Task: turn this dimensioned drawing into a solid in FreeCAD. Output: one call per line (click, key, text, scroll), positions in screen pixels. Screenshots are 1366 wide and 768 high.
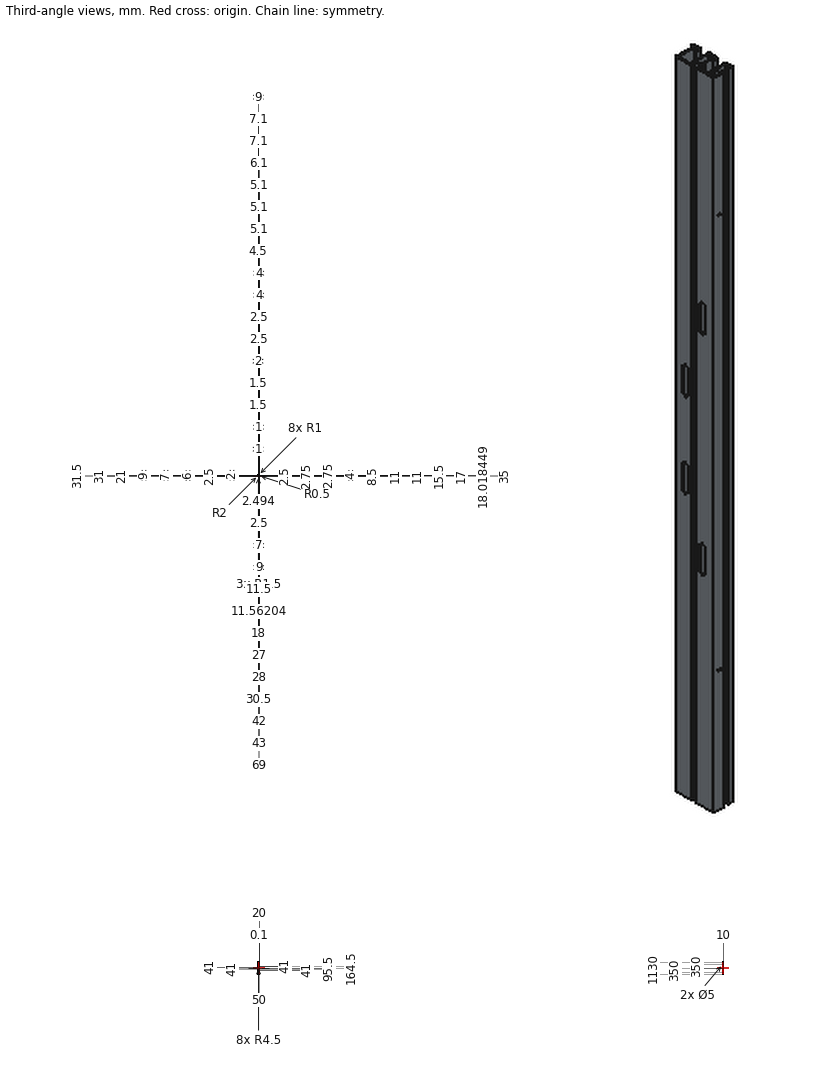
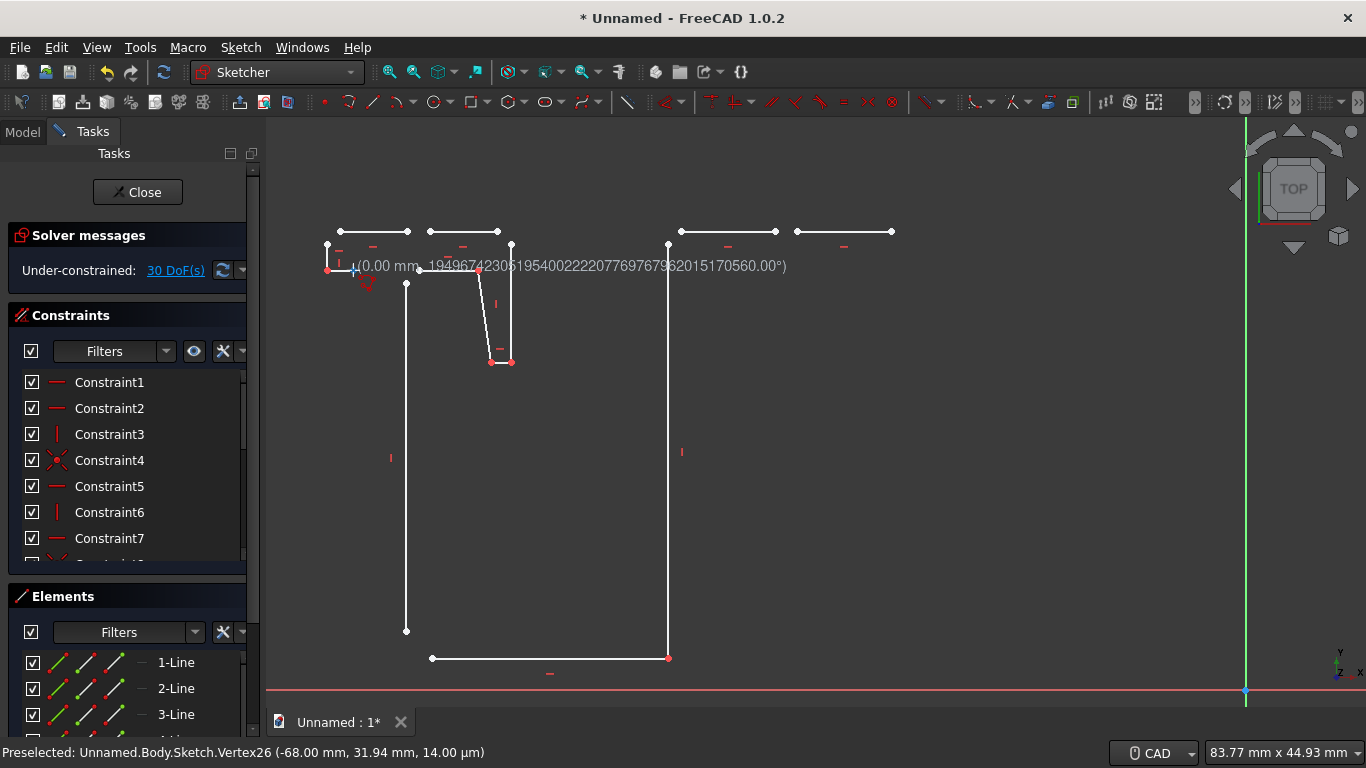
click(366, 283)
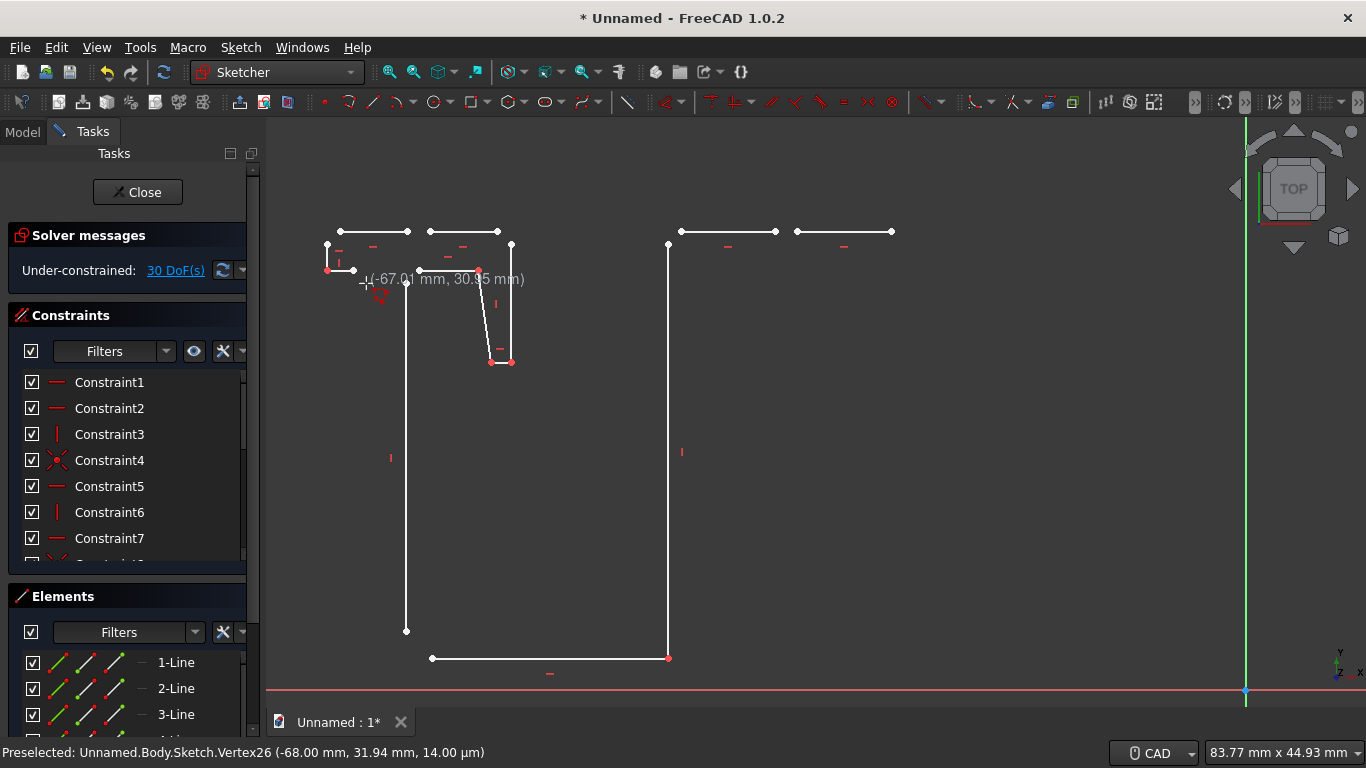
scroll(669, 313, down, 2)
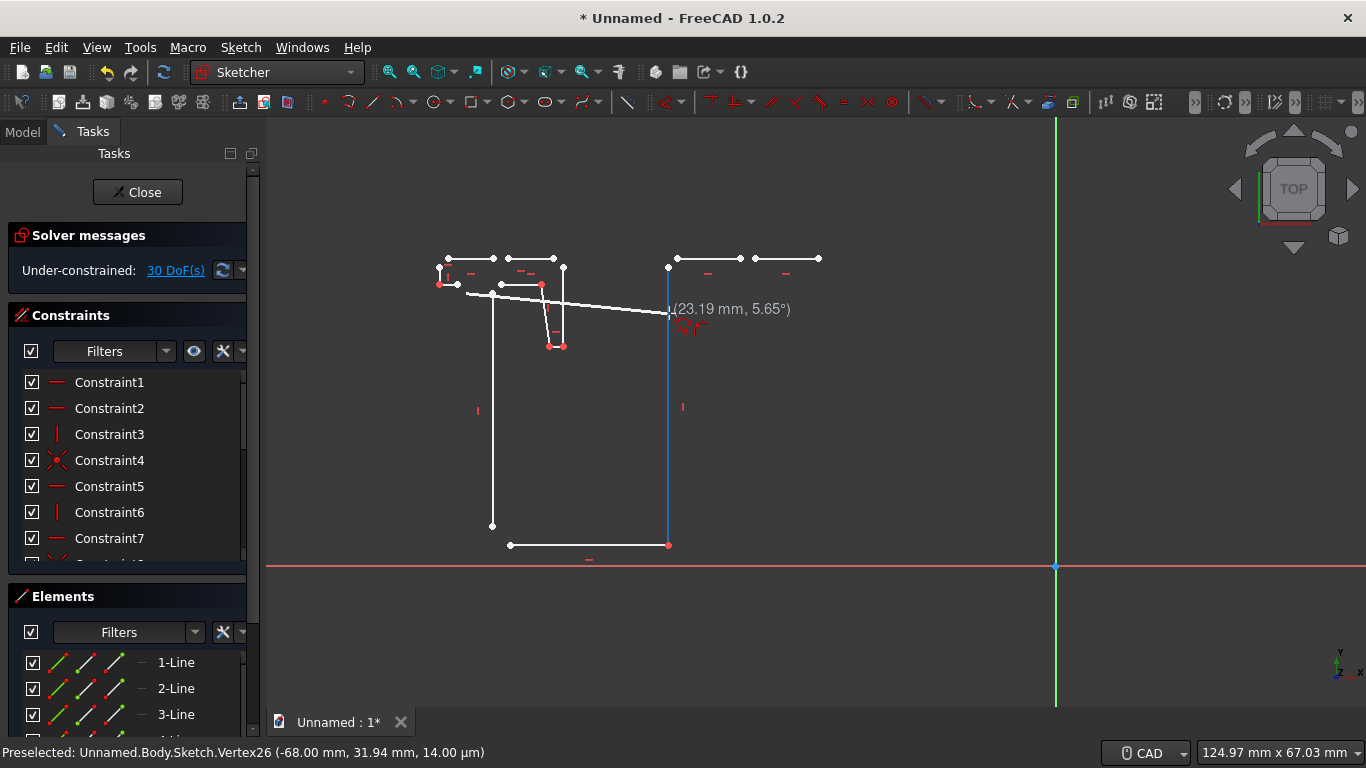
click(466, 566)
click(713, 557)
click(713, 544)
click(691, 544)
click(691, 491)
click(809, 491)
click(809, 544)
click(787, 544)
click(787, 566)
click(1056, 566)
click(1047, 405)
click(1034, 405)
click(1034, 430)
click(955, 430)
click(955, 293)
right_click(955, 293)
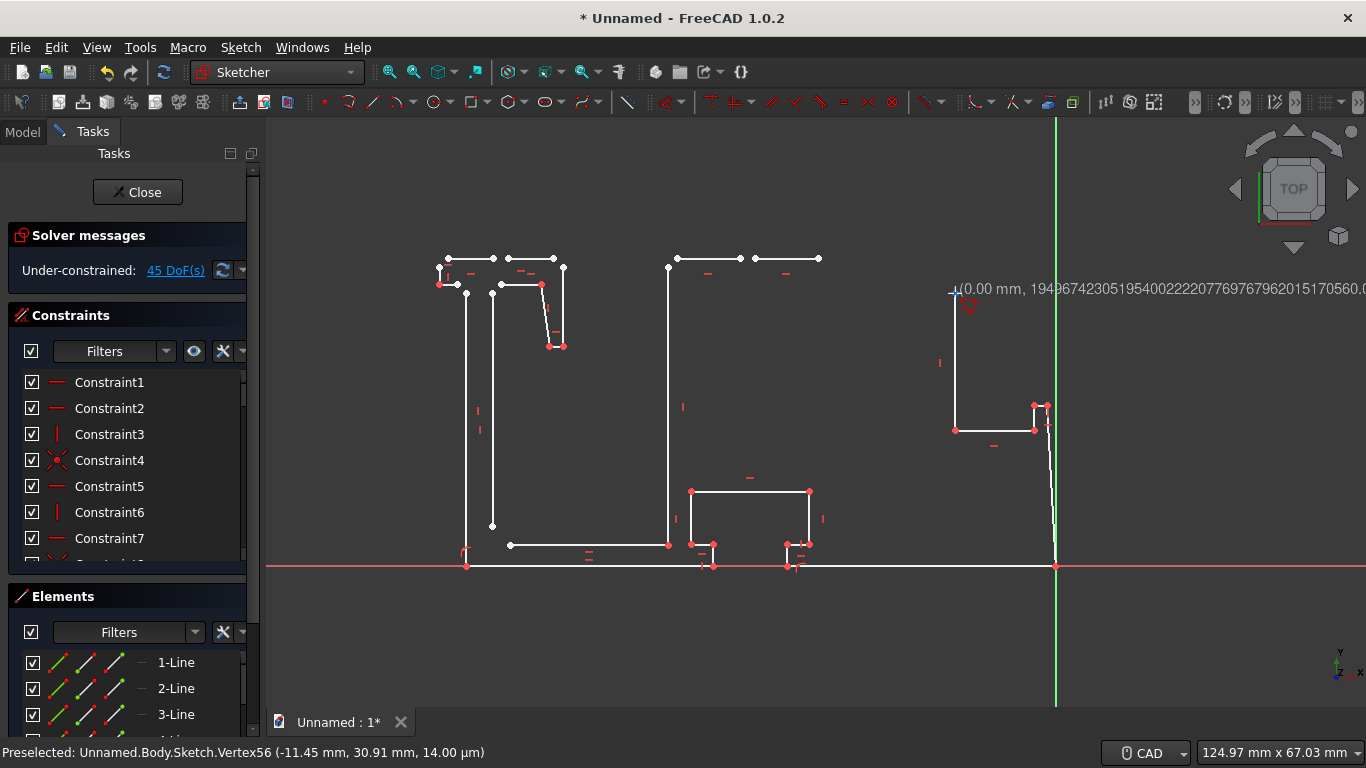
scroll(963, 284, up, 2)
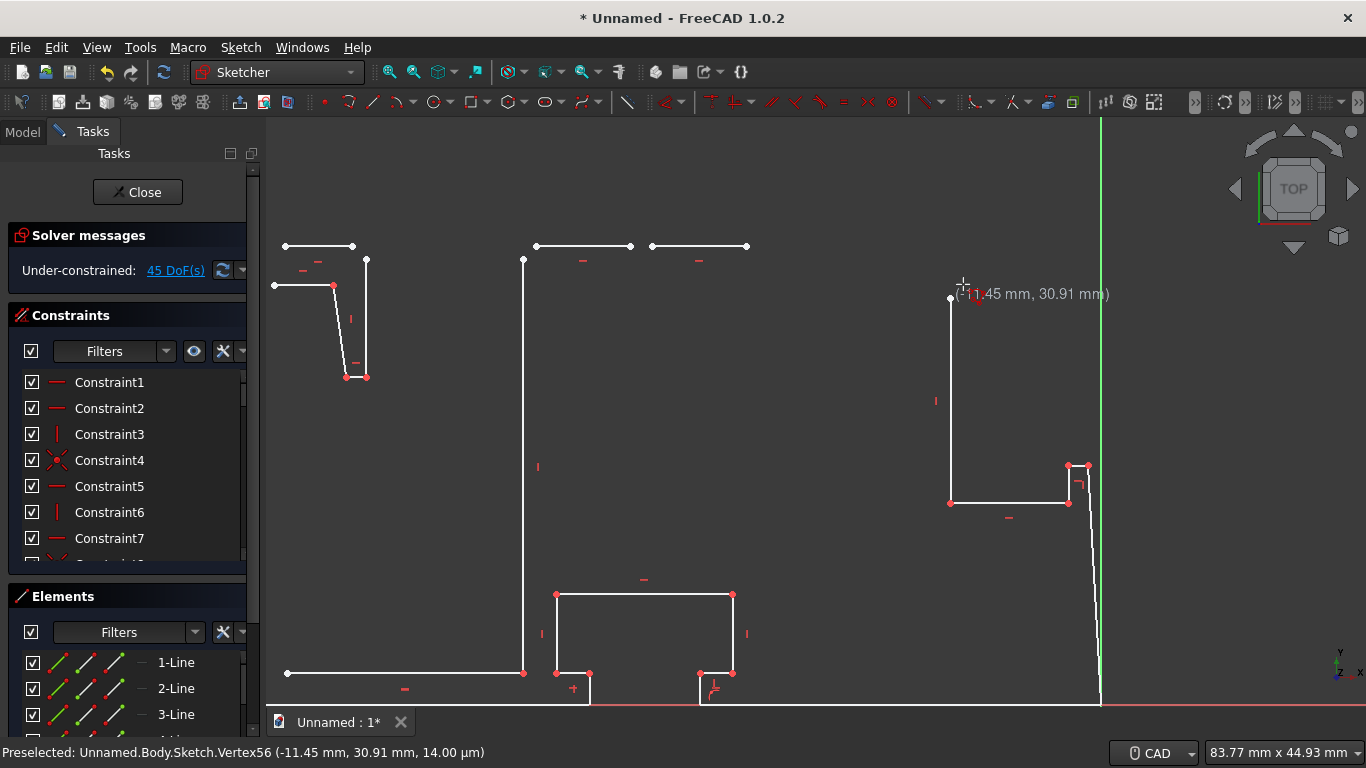
click(963, 284)
click(1016, 284)
click(1016, 317)
click(1068, 317)
click(1068, 353)
click(1101, 353)
click(1092, 245)
click(1021, 245)
right_click(1021, 245)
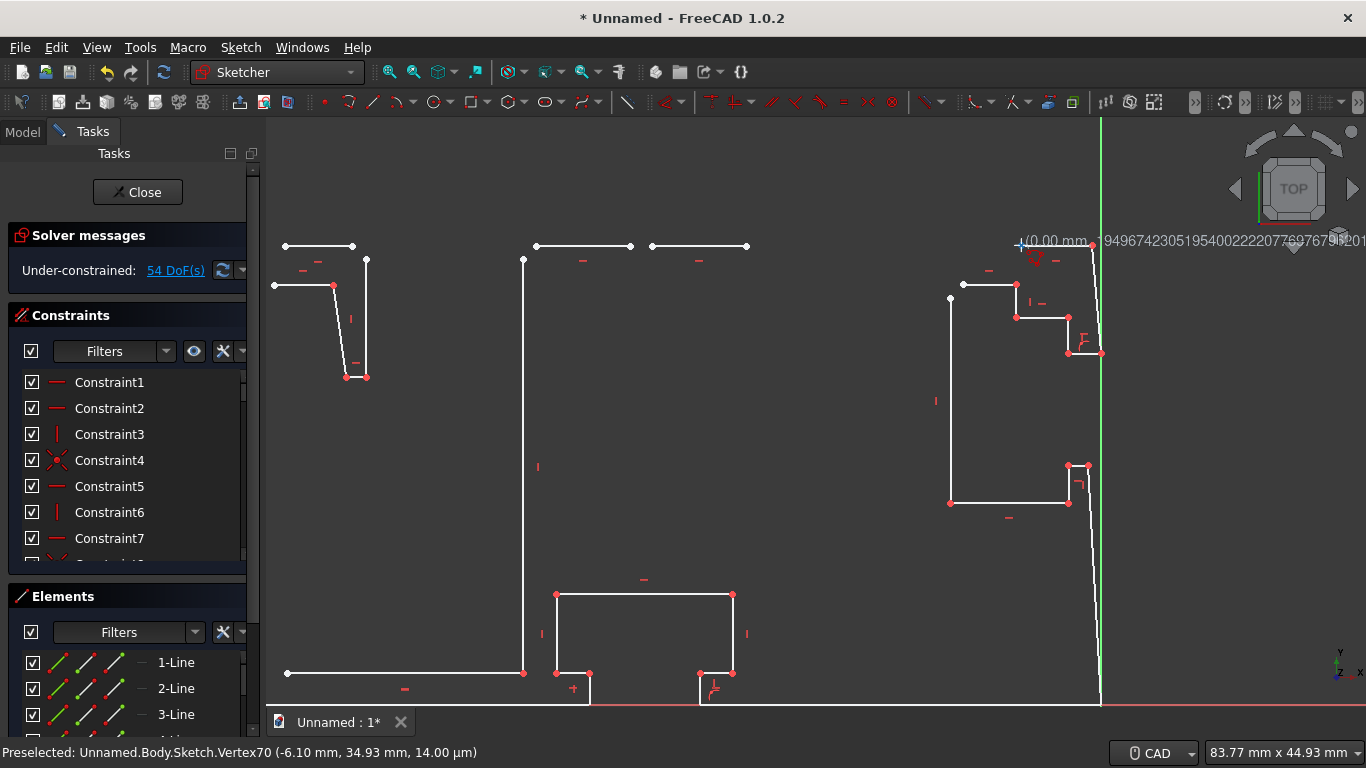
click(374, 102)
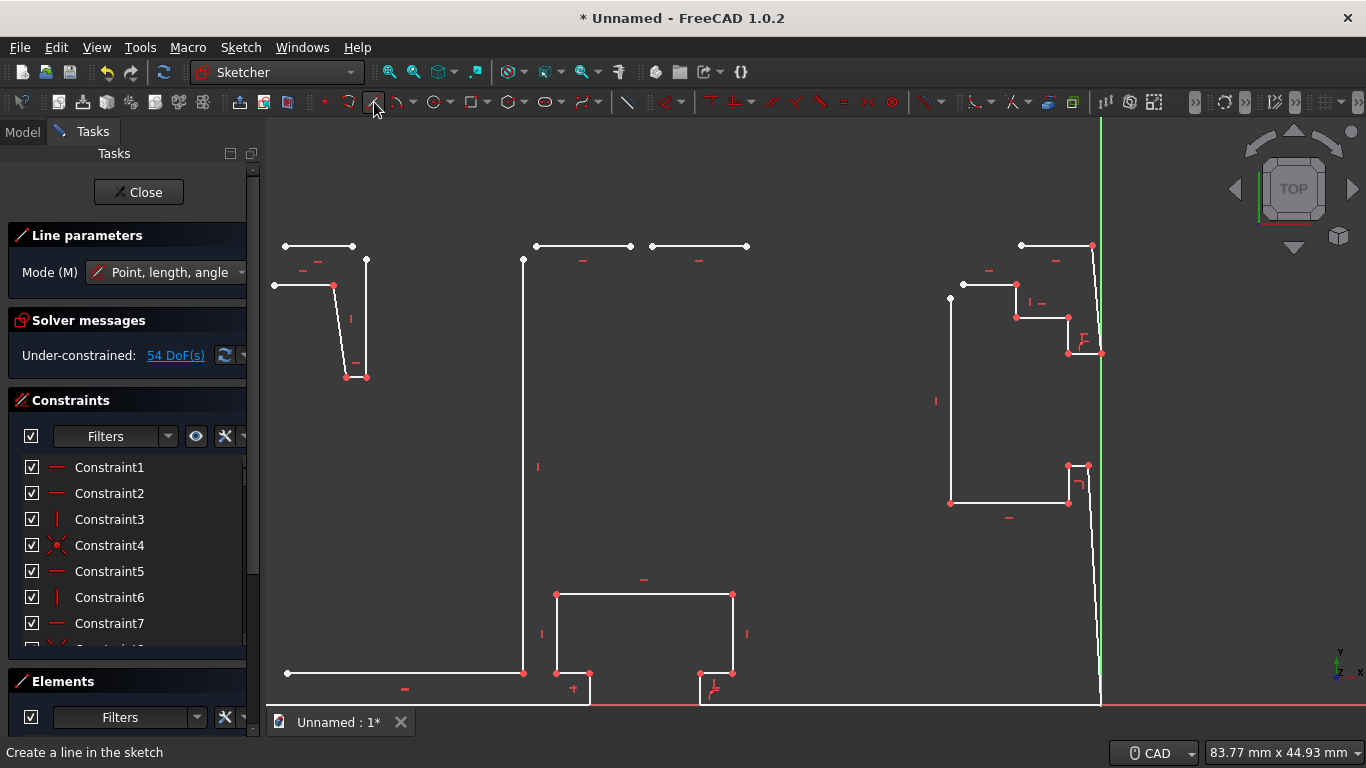
click(997, 245)
click(930, 245)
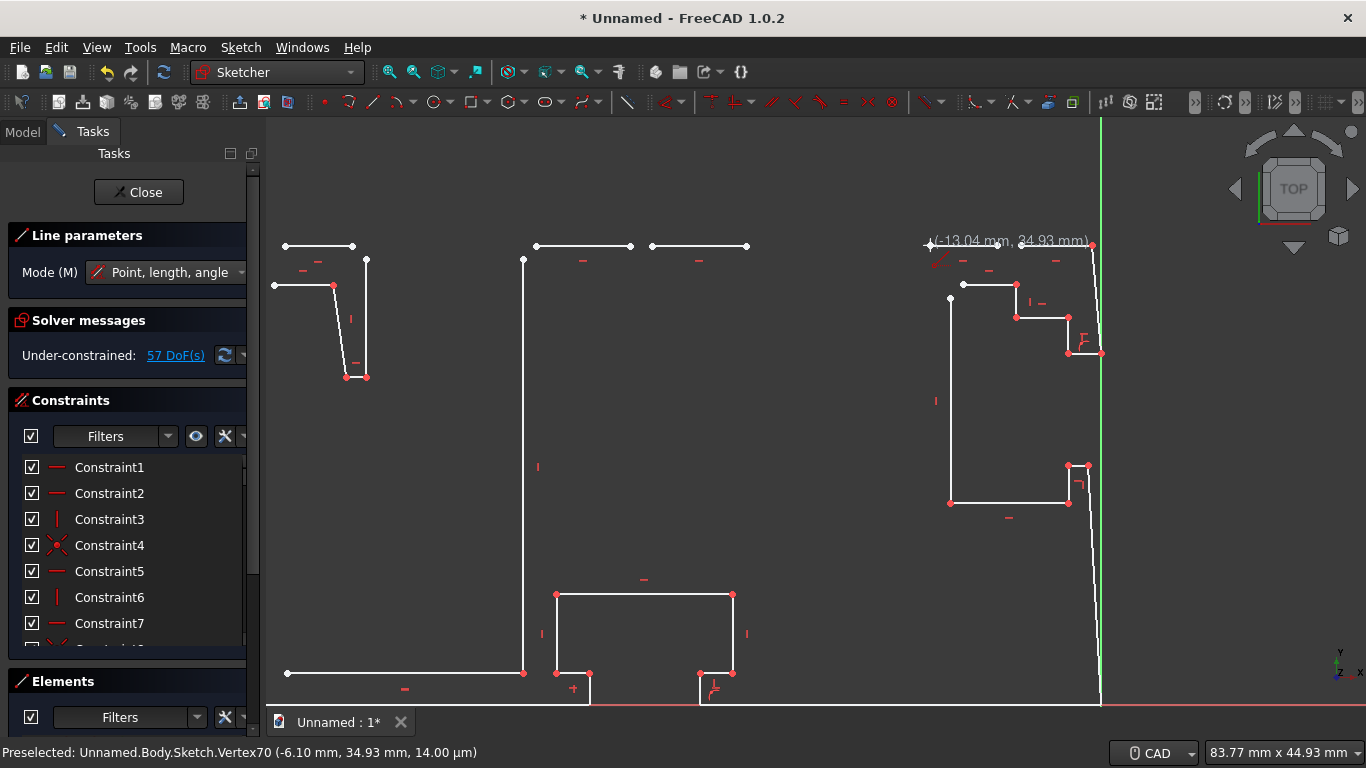
key(g)
key(m)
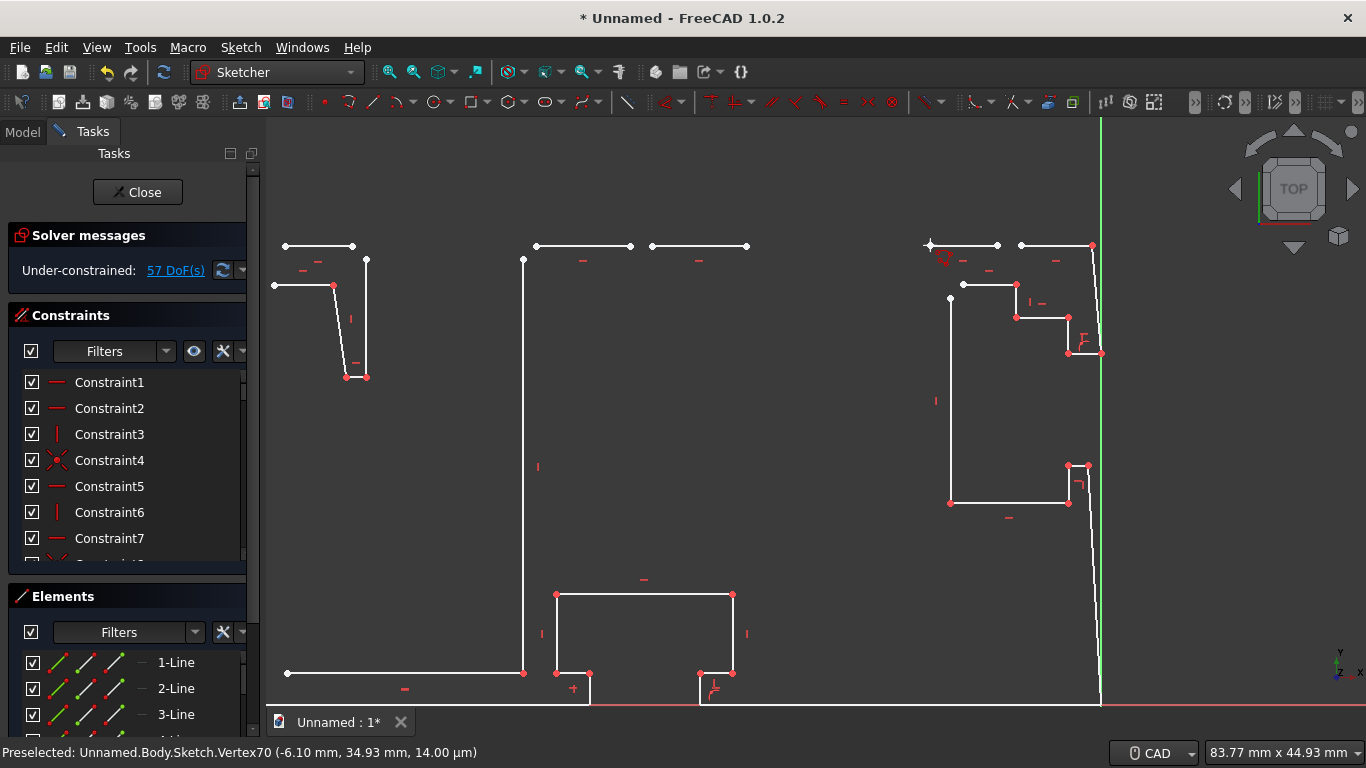
click(917, 258)
click(917, 672)
click(766, 672)
click(766, 560)
click(694, 508)
click(694, 284)
click(727, 284)
click(740, 376)
click(760, 376)
click(760, 258)
right_click(760, 258)